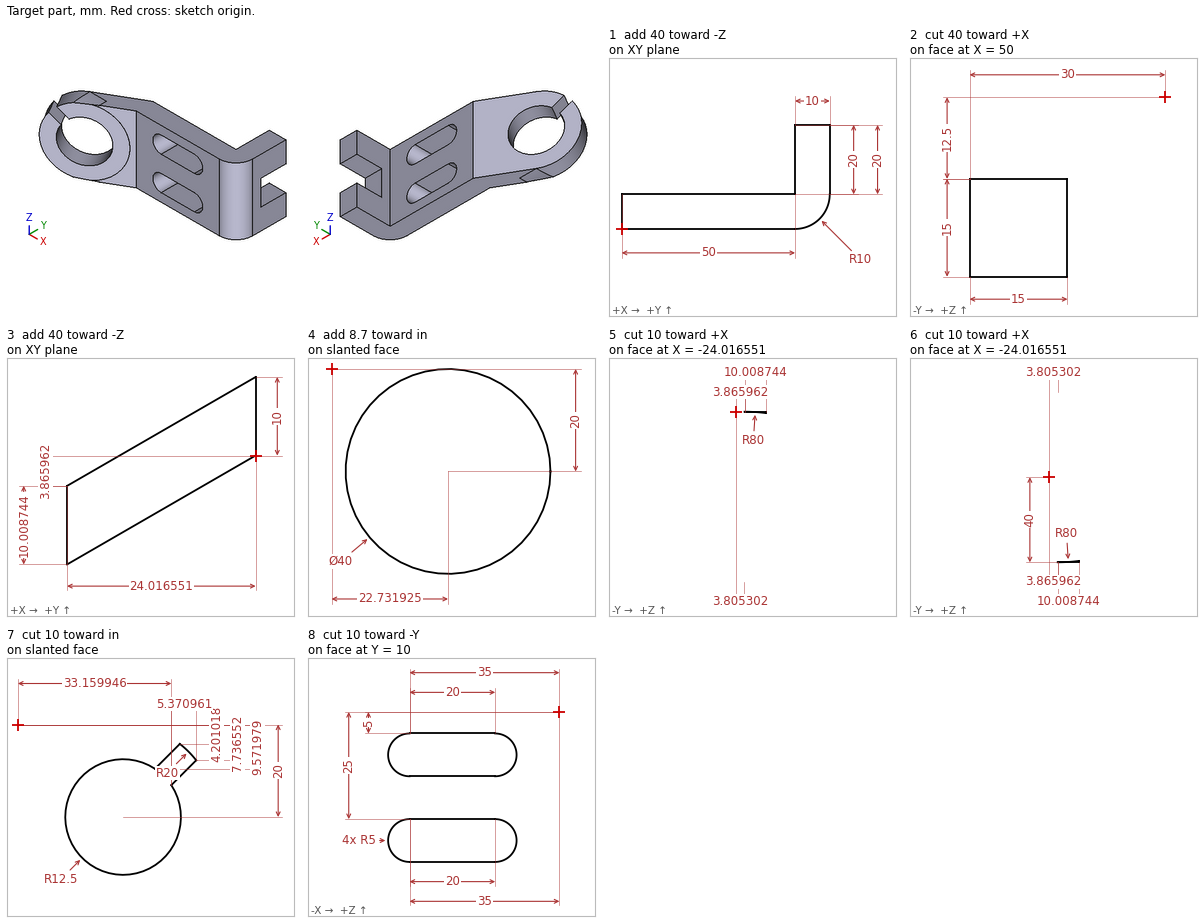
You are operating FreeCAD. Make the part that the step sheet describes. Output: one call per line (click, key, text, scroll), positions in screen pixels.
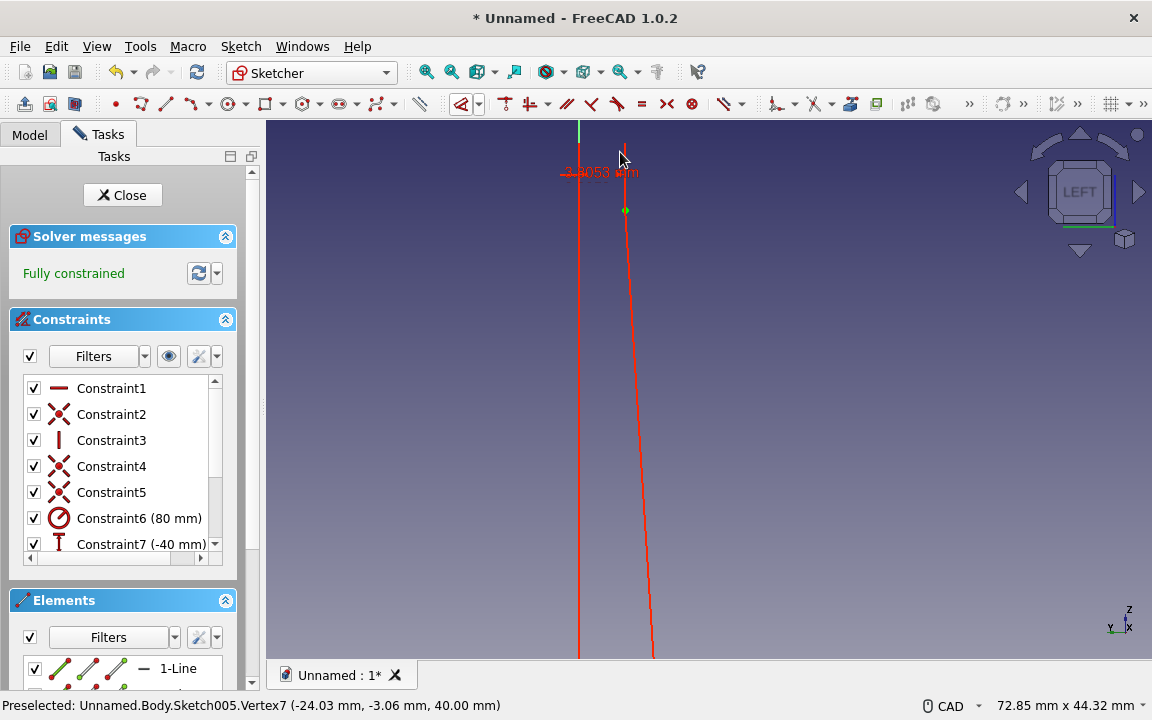
click(123, 195)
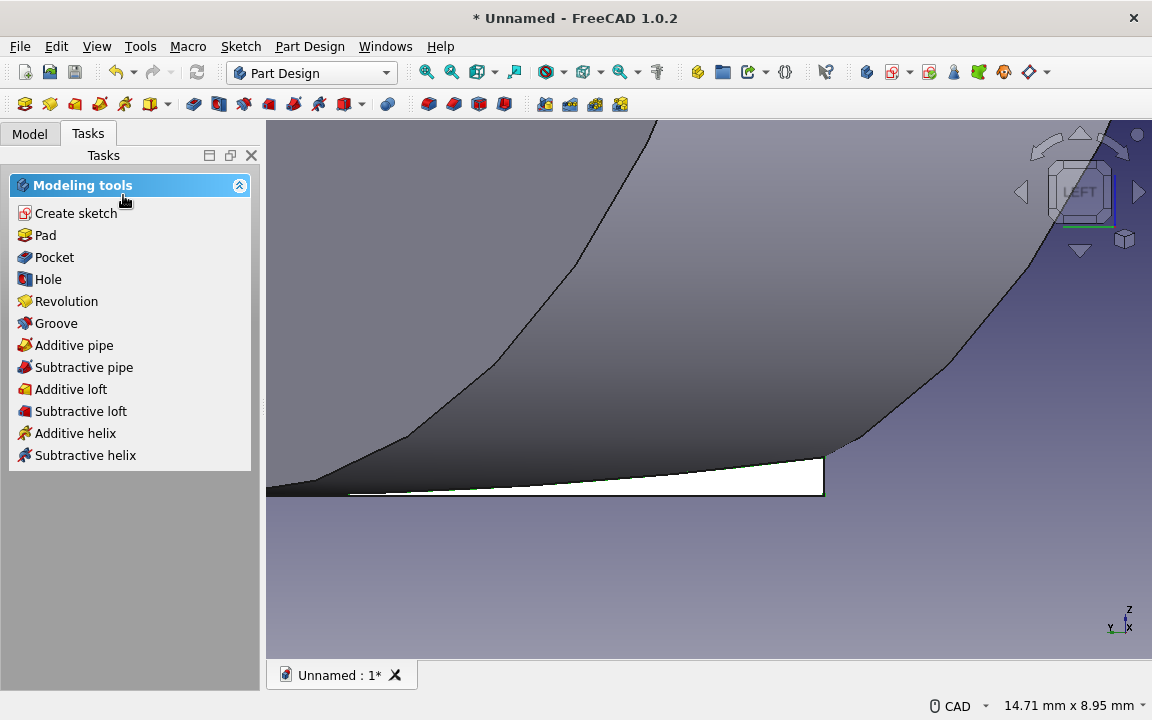
click(194, 104)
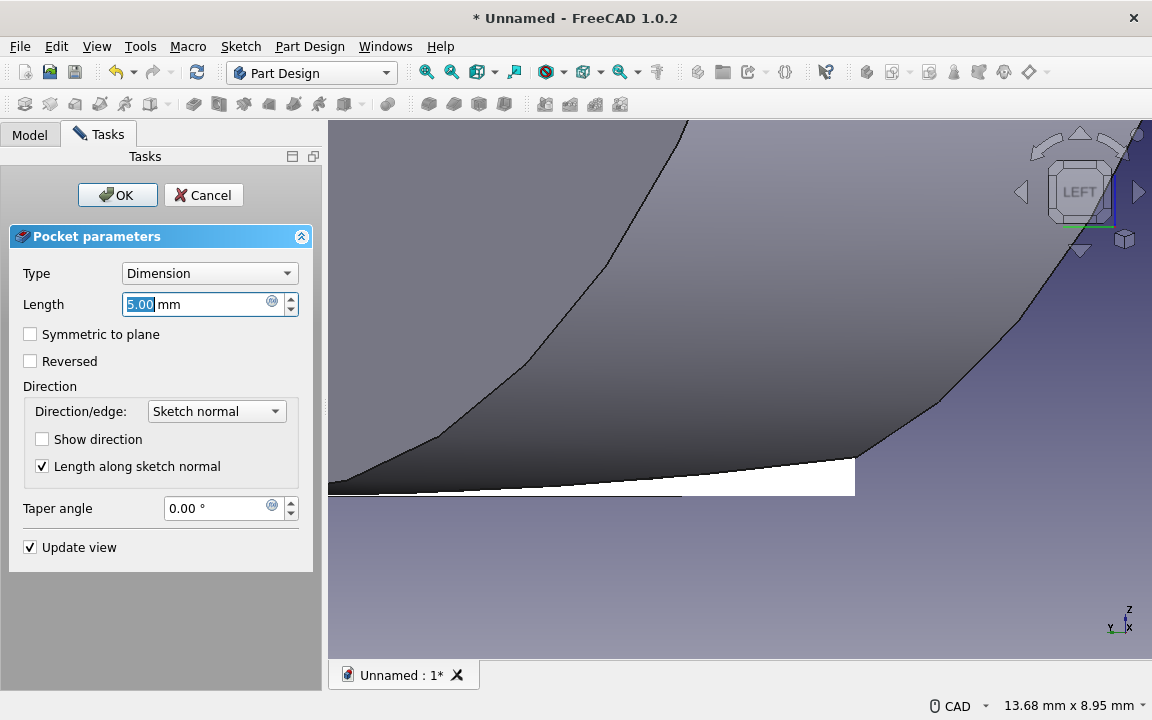
text(10)
key(Tab)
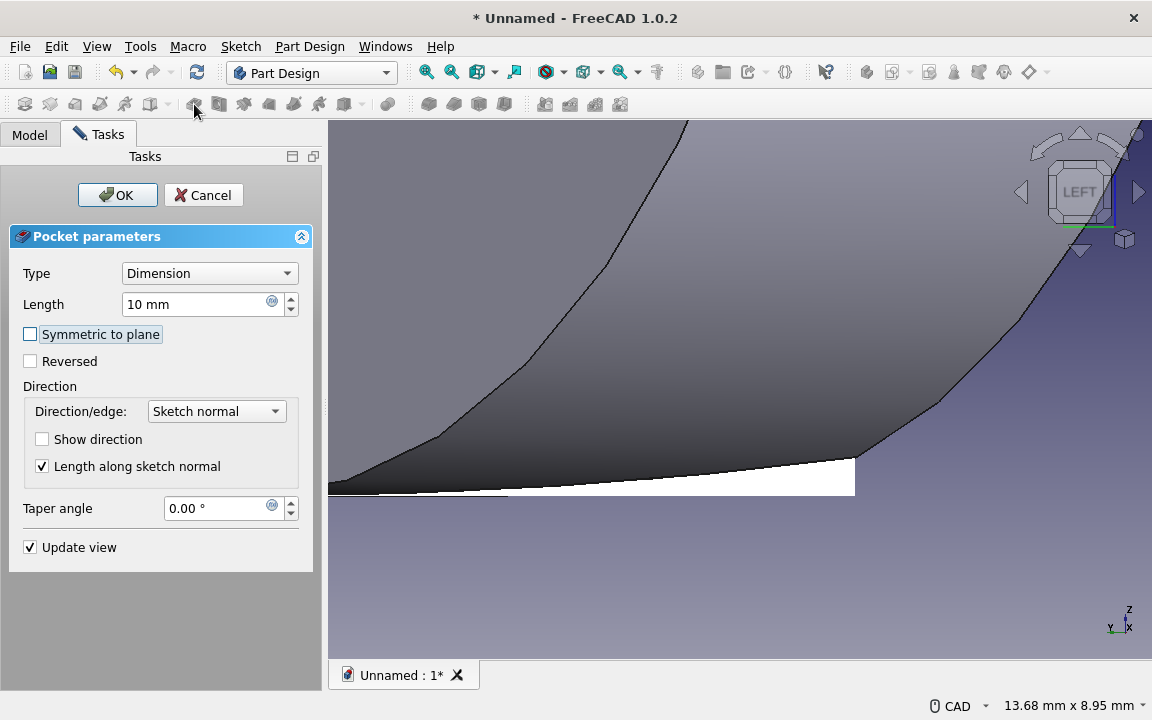
click(118, 195)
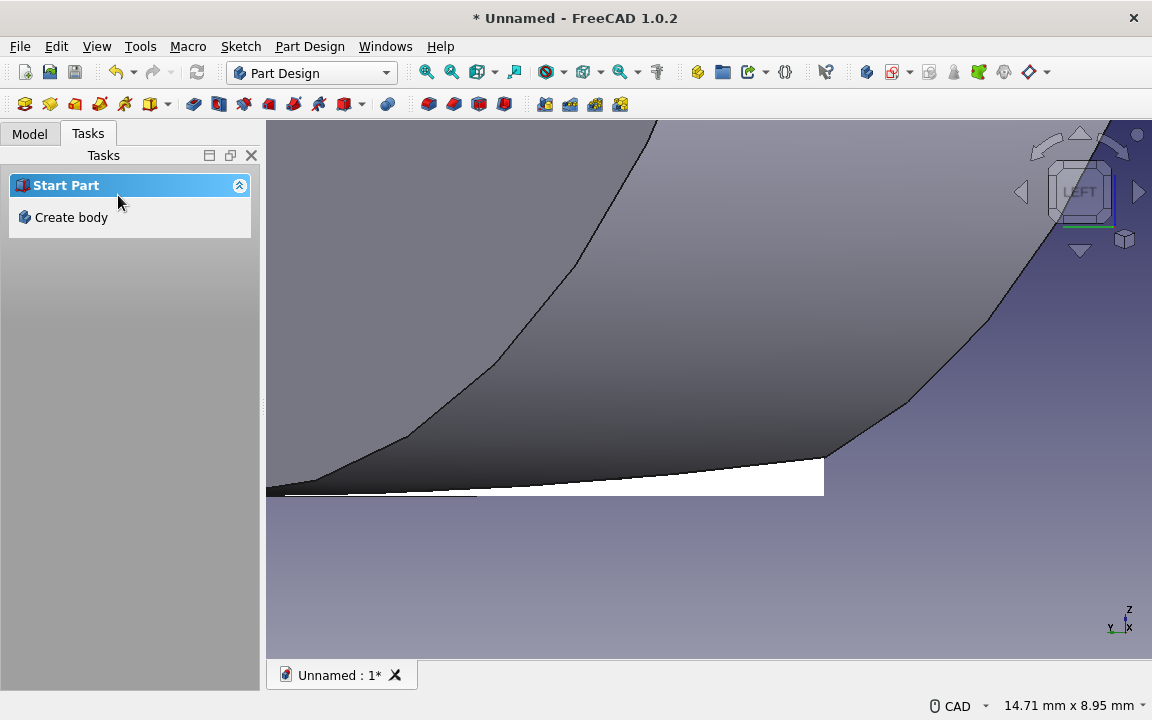
click(427, 72)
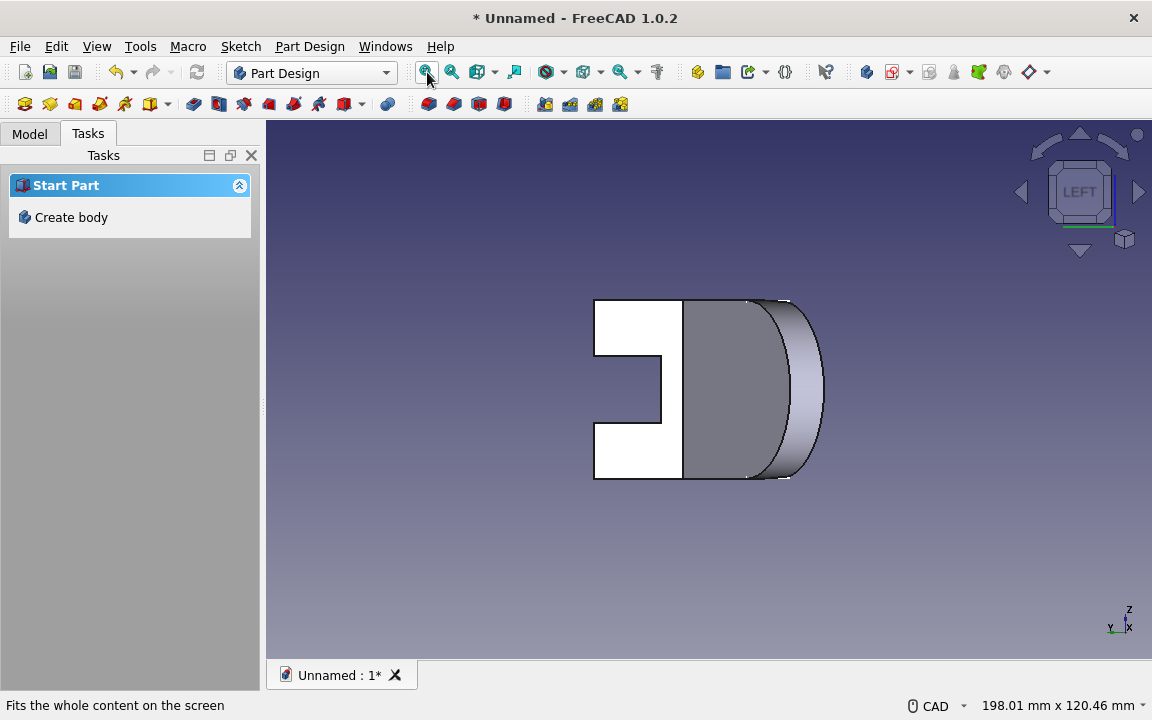
click(737, 388)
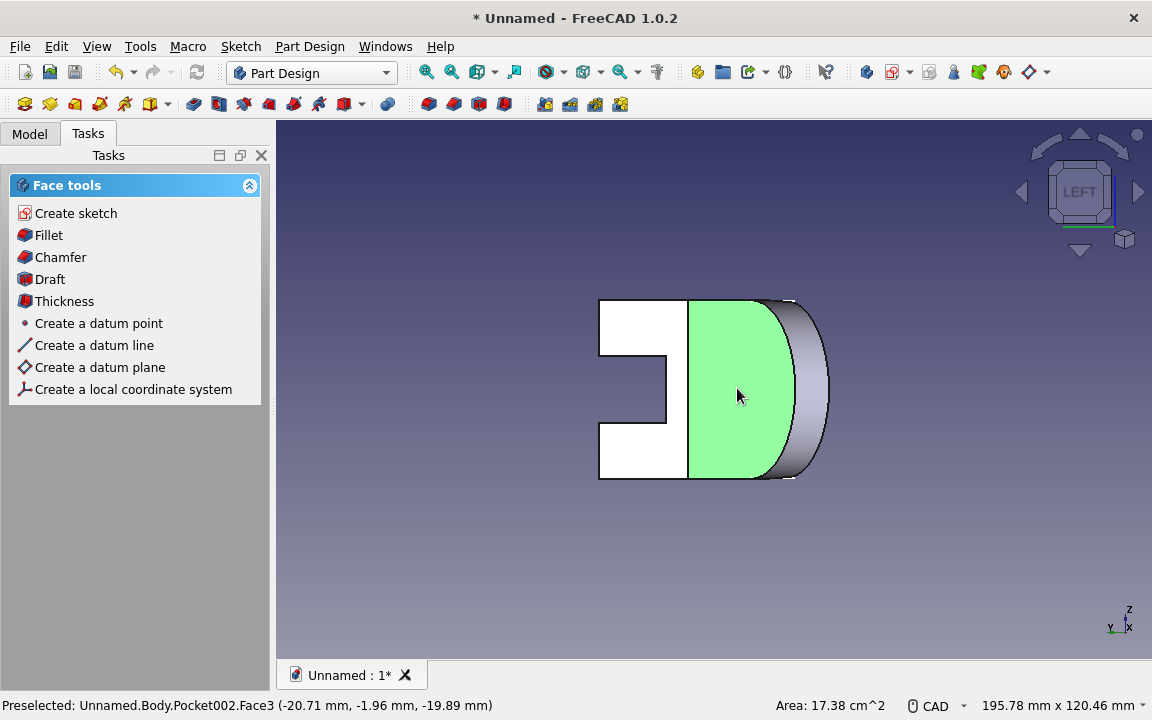
click(892, 72)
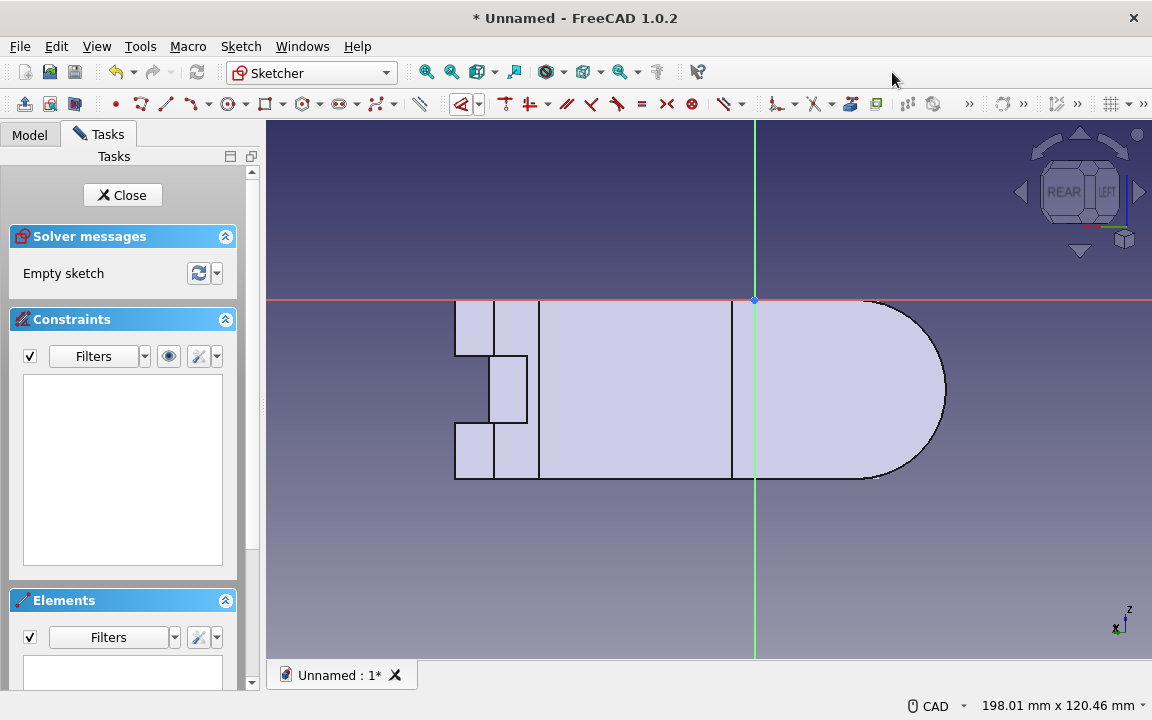
key(q)
key(s)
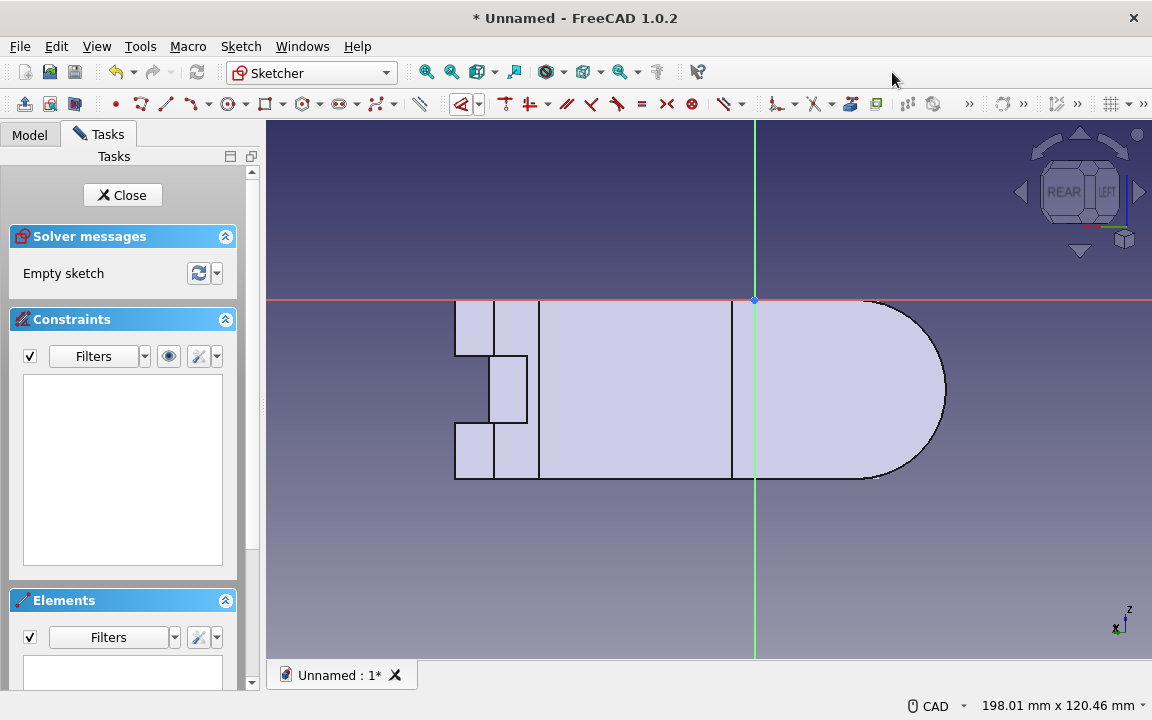
scroll(958, 350, up, 5)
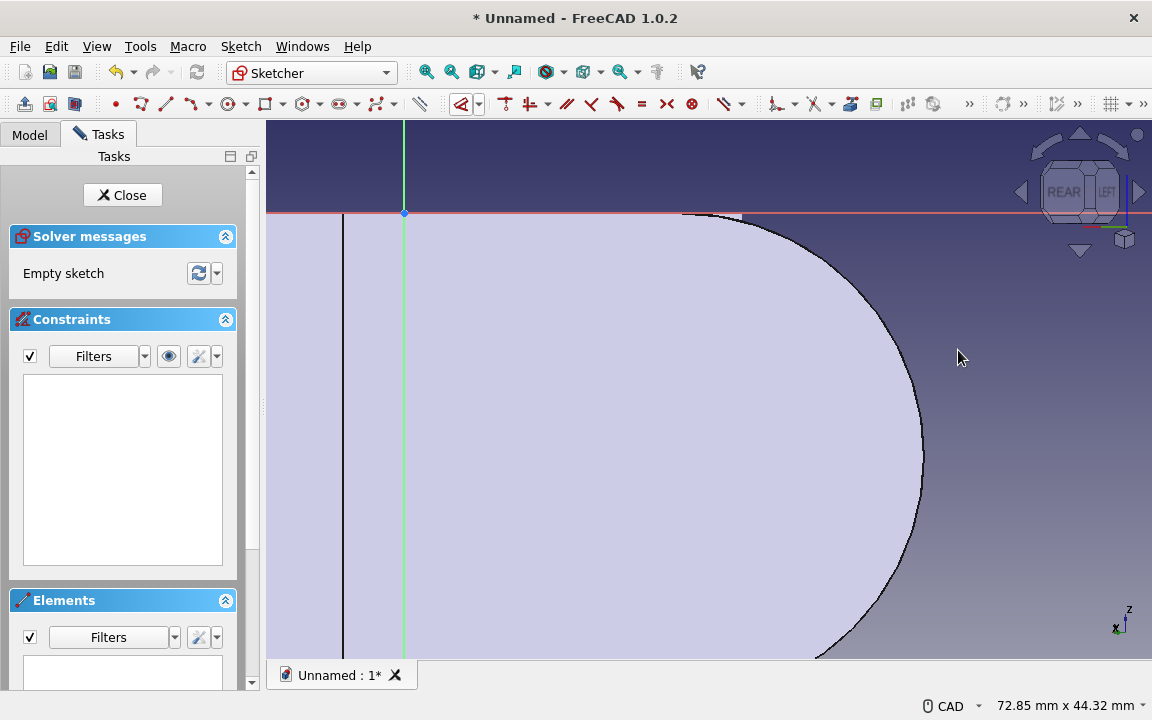
click(166, 104)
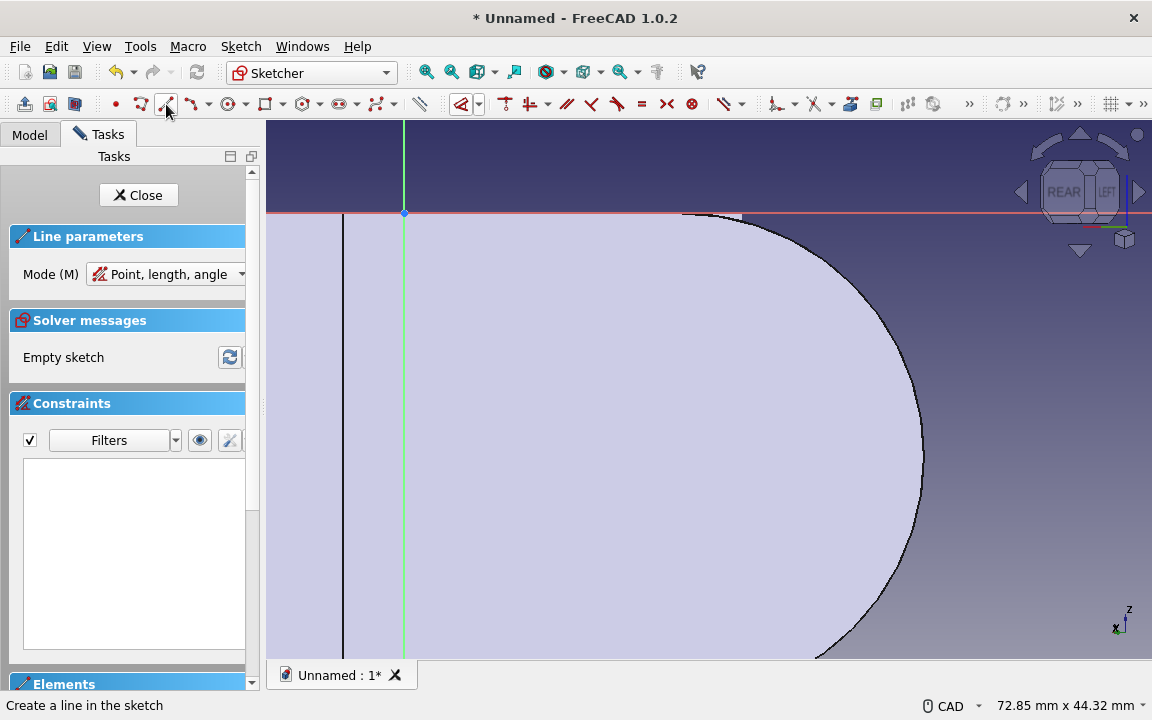
click(808, 373)
click(873, 307)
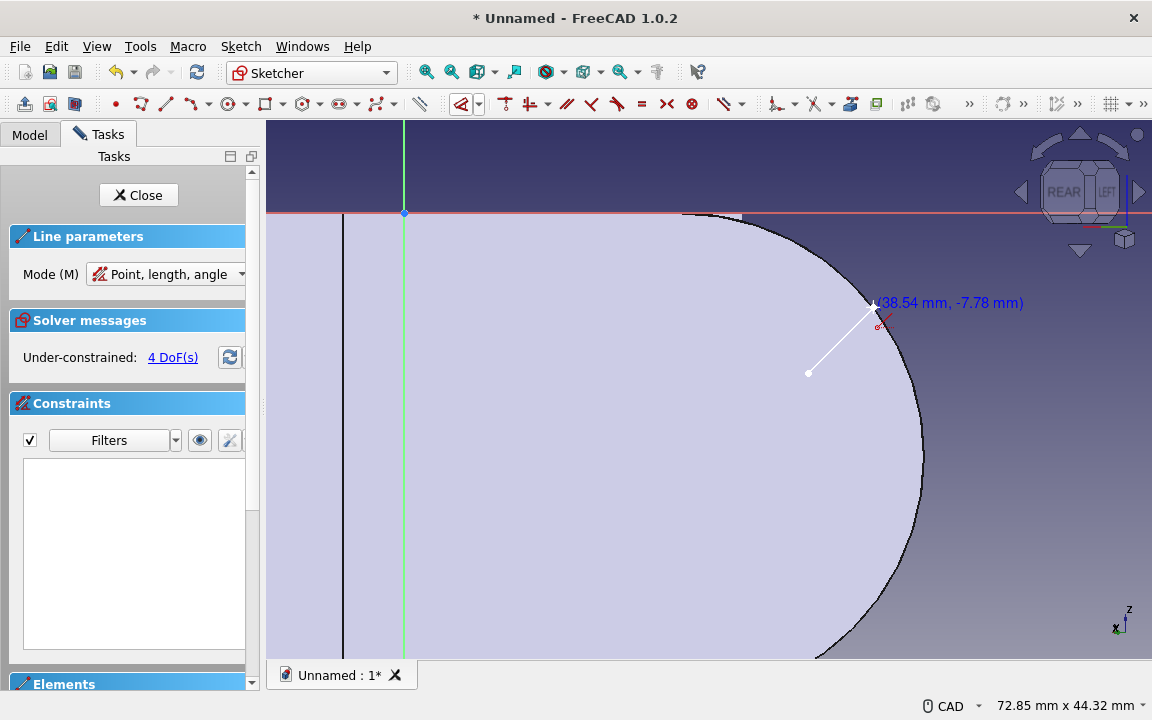
click(830, 264)
click(765, 330)